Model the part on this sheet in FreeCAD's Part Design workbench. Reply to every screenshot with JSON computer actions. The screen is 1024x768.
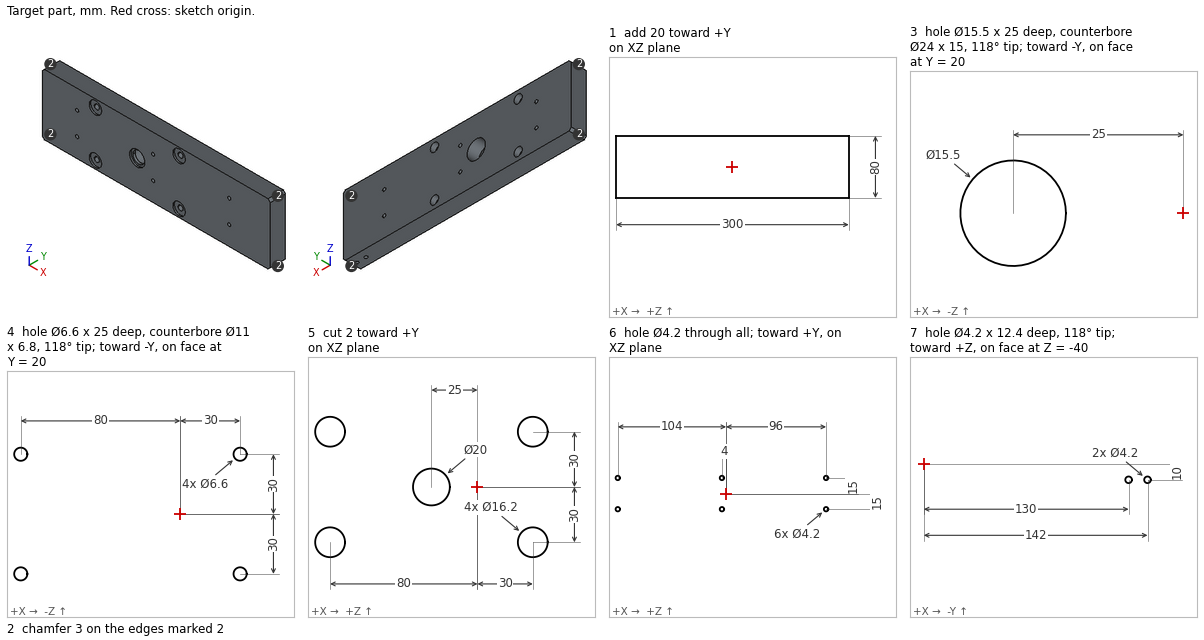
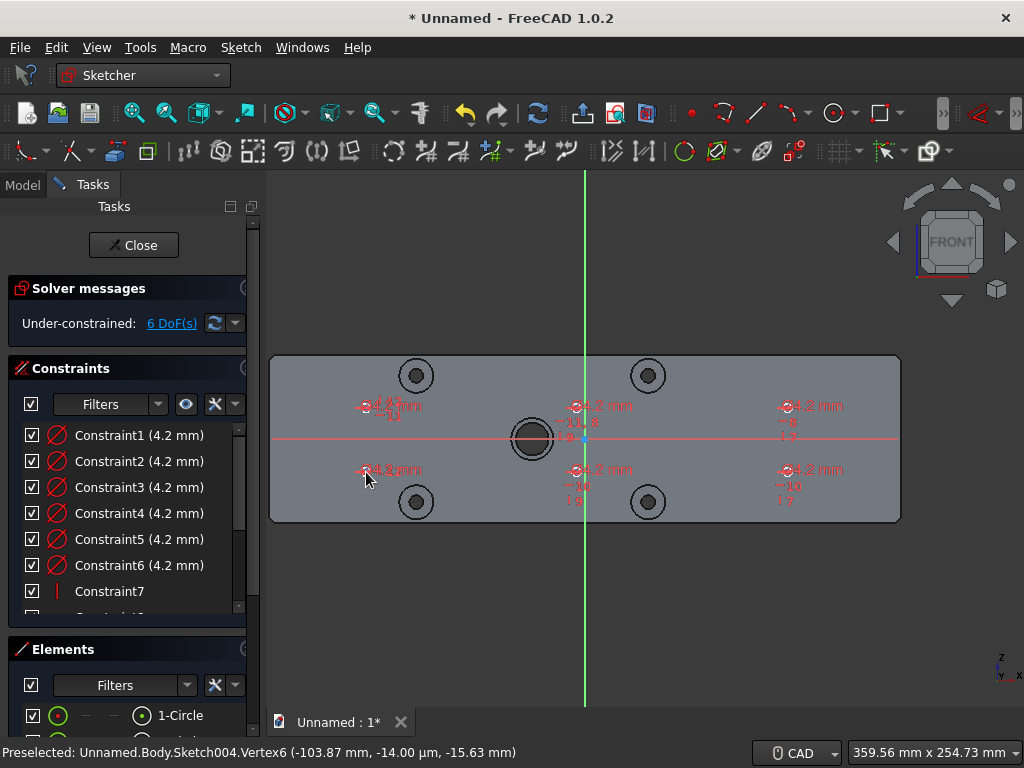
{"action": "left_click", "coordinate": [577, 472]}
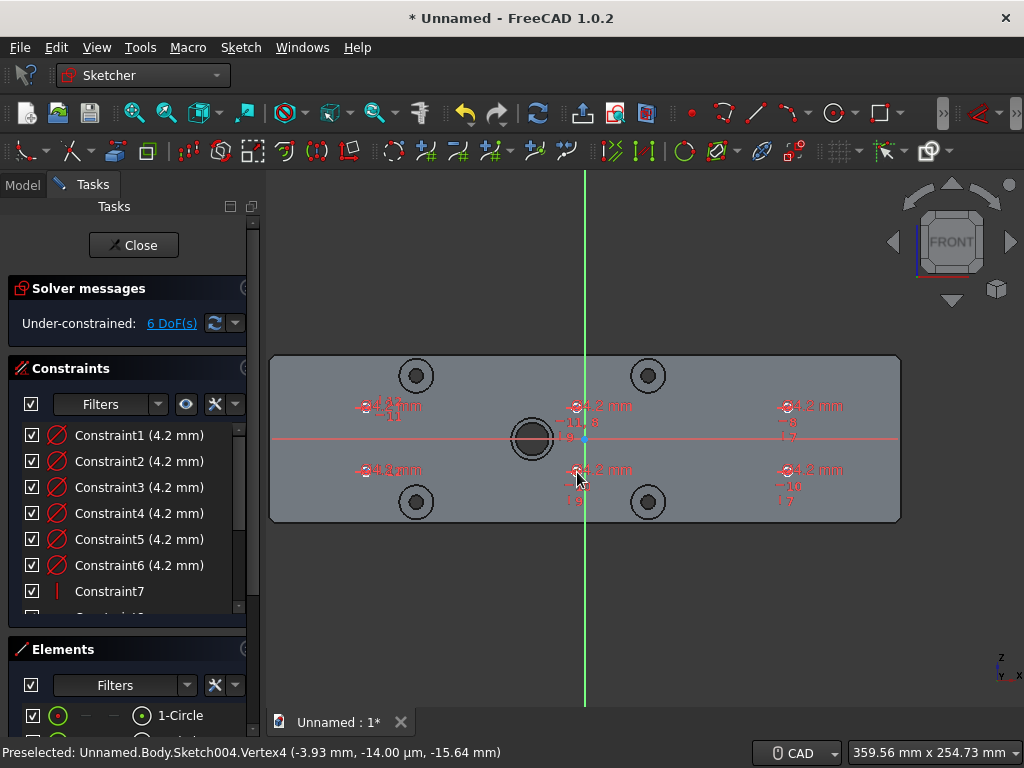
{"action": "left_click", "coordinate": [366, 472]}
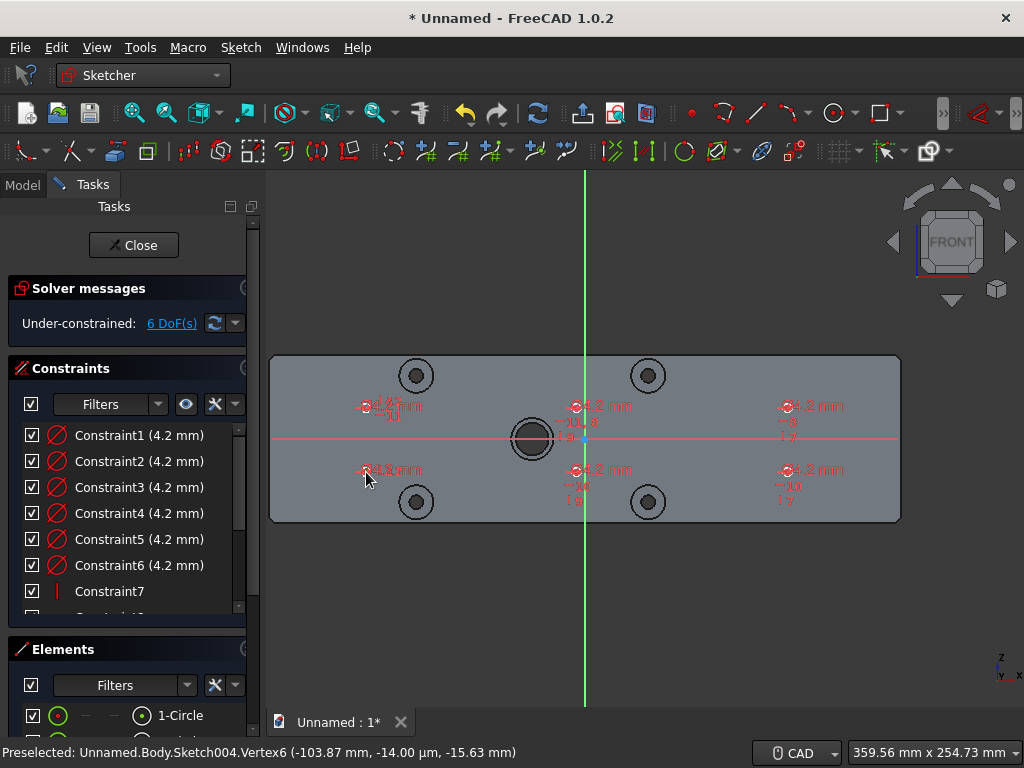
{"action": "key", "text": "h"}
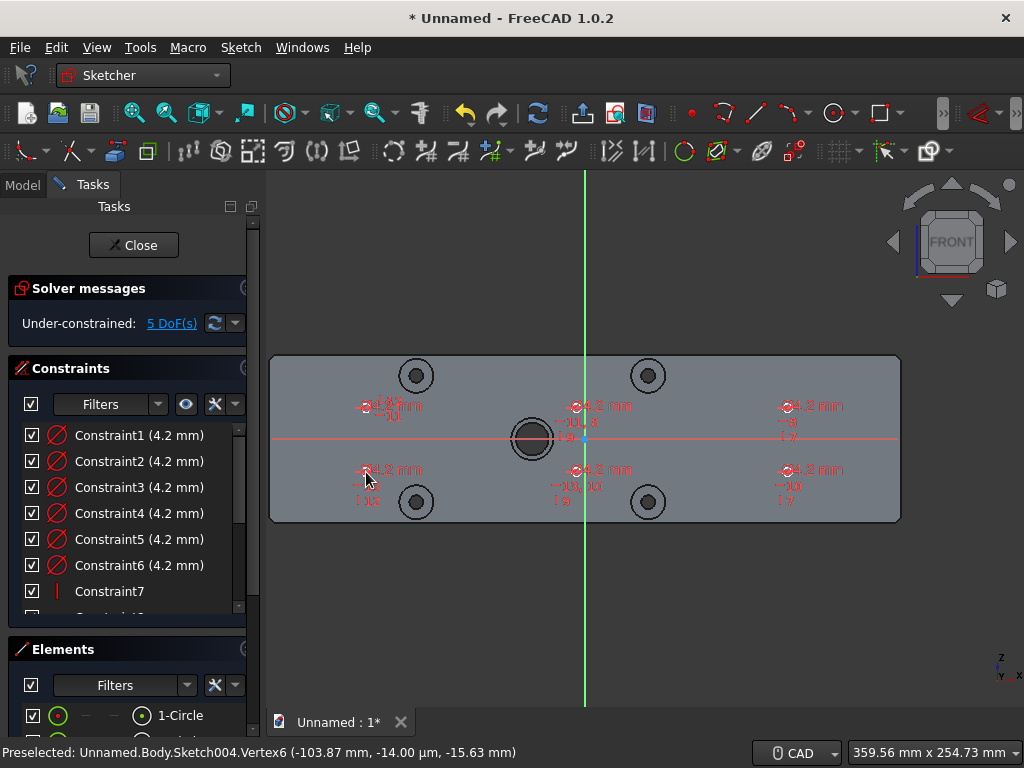
{"action": "left_click", "coordinate": [978, 114]}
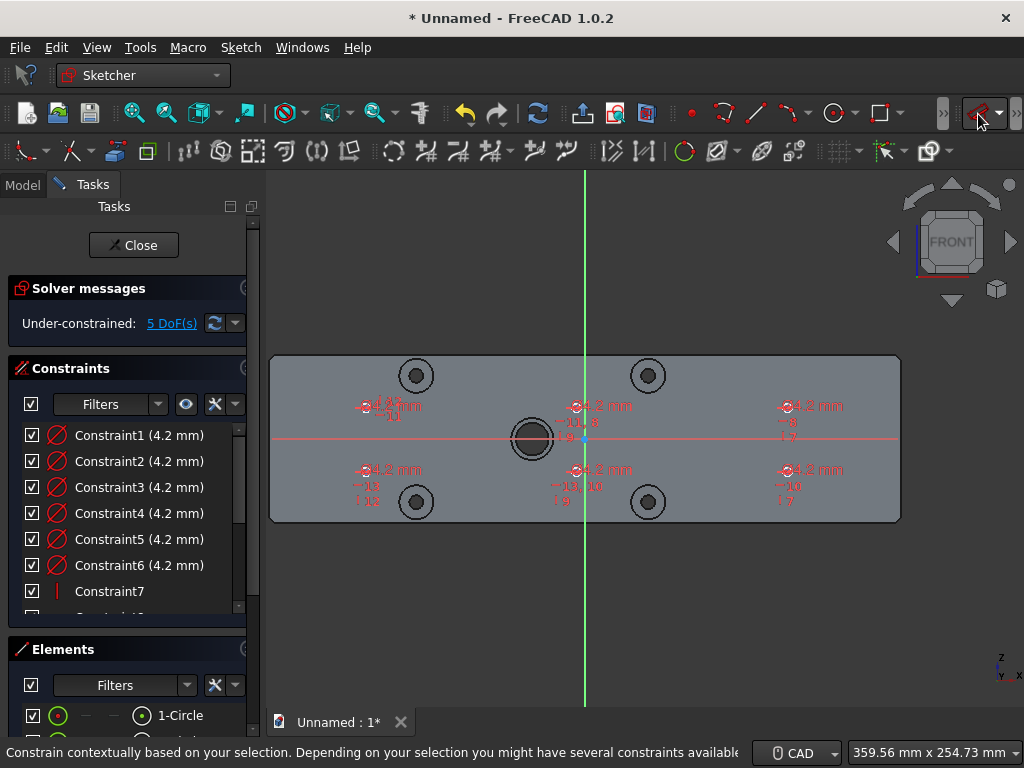
{"action": "scroll", "coordinate": [577, 408], "scroll_direction": "up", "scroll_amount": 8}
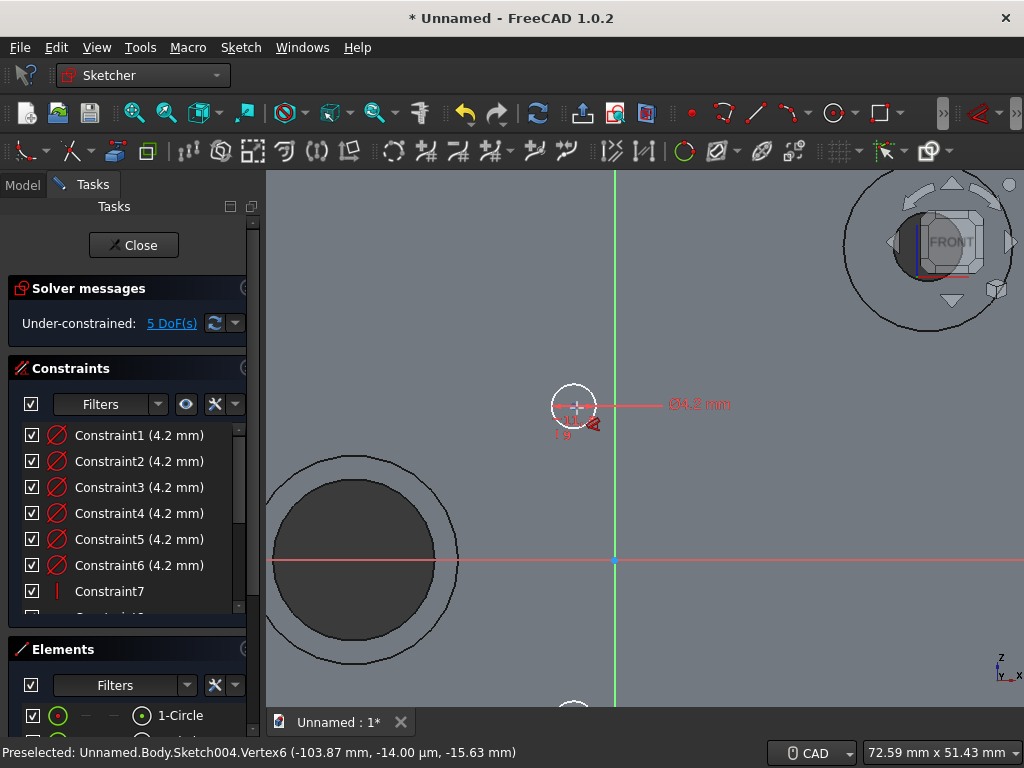
{"action": "left_click", "coordinate": [574, 406]}
{"action": "left_click", "coordinate": [594, 372]}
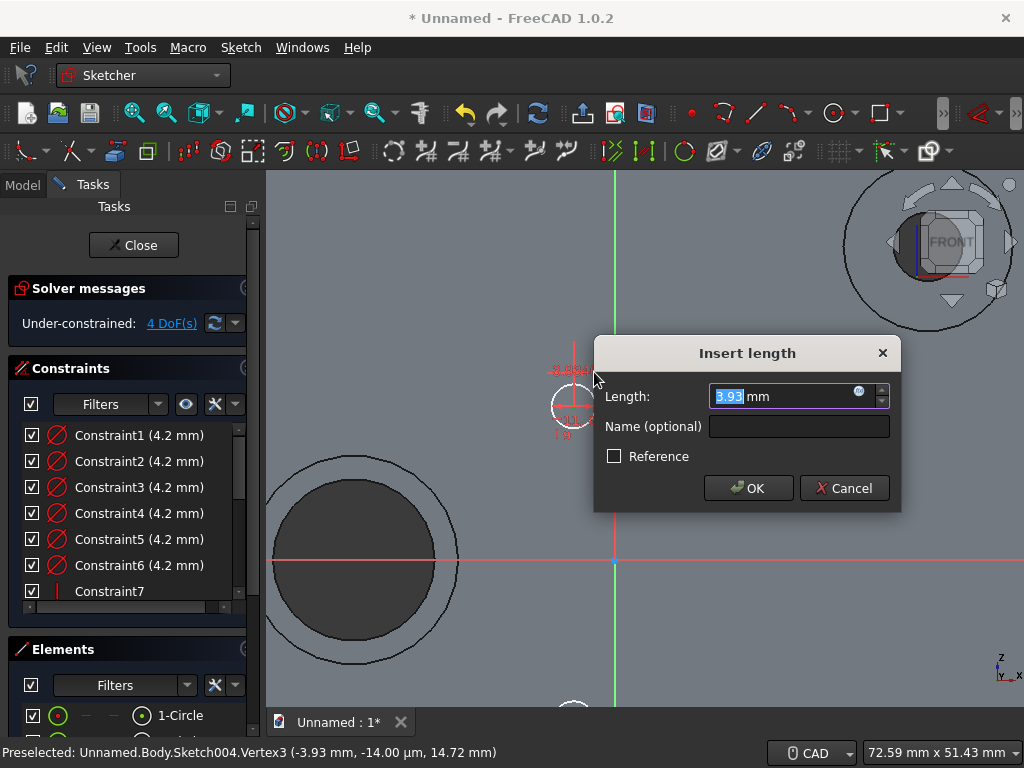
{"action": "type", "text": "4"}
{"action": "key", "text": "Return"}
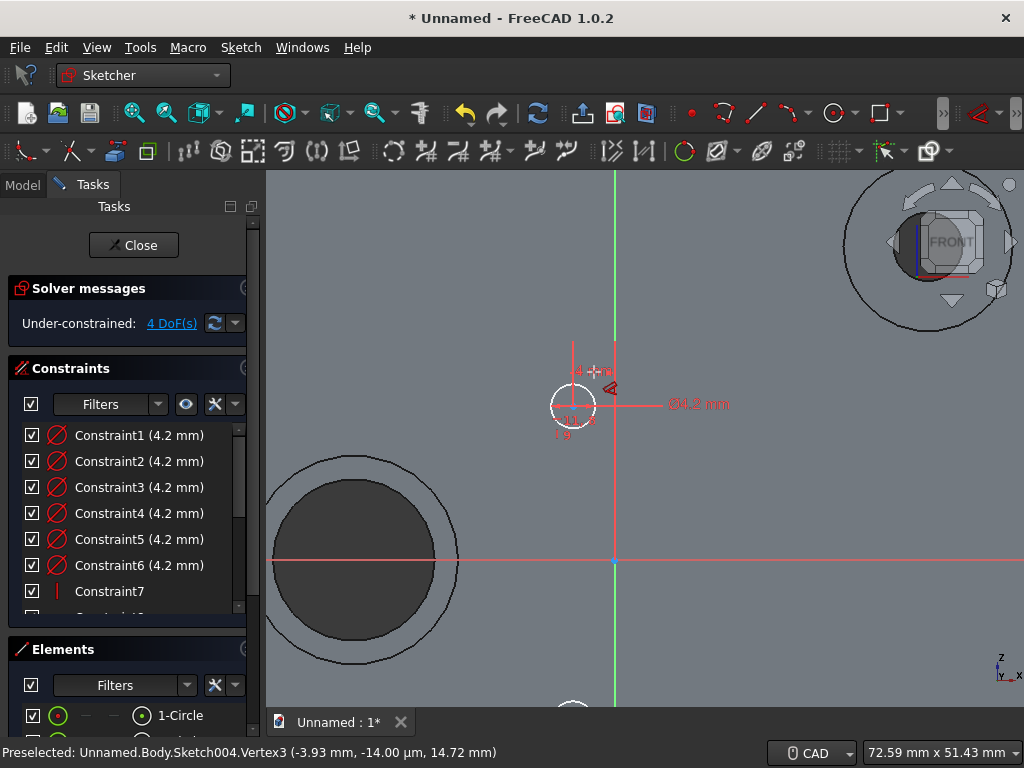
{"action": "scroll", "coordinate": [577, 408], "scroll_direction": "down", "scroll_amount": 8}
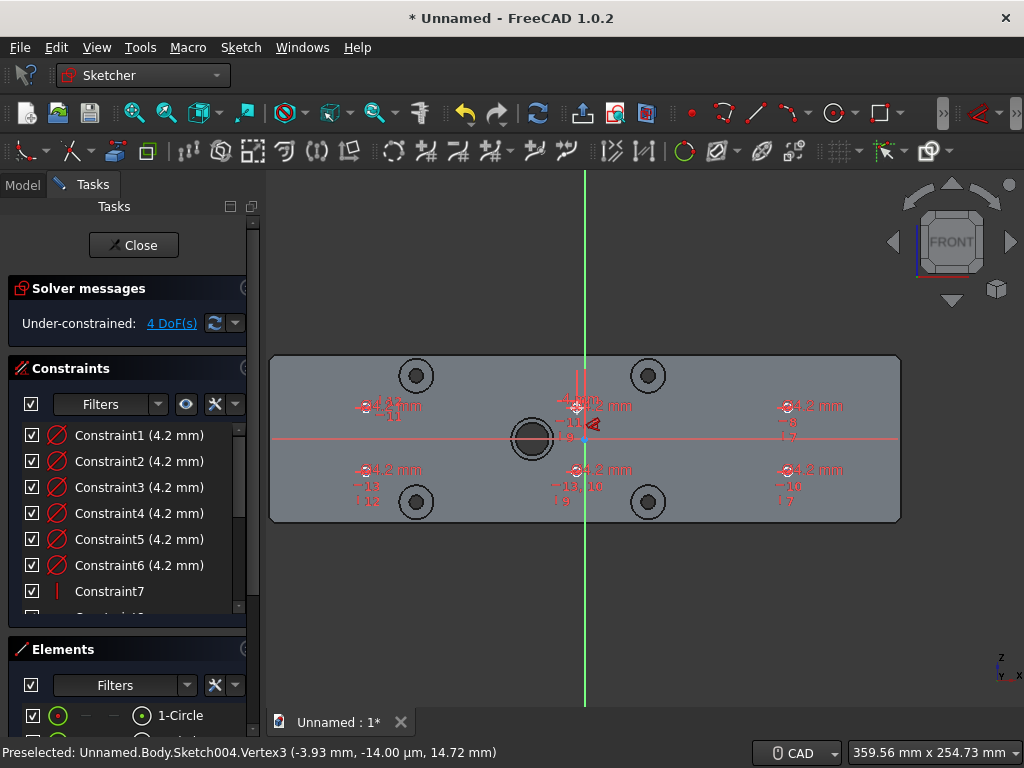
{"action": "left_click", "coordinate": [787, 408]}
{"action": "left_click", "coordinate": [686, 374]}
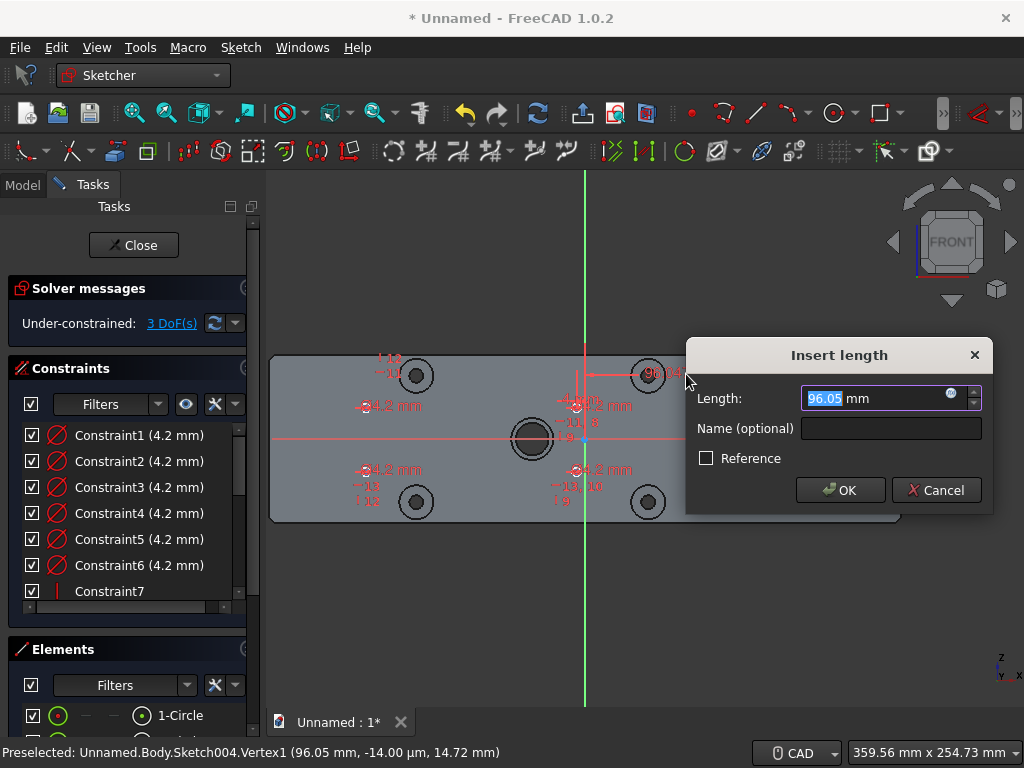
{"action": "type", "text": "96"}
{"action": "key", "text": "Return"}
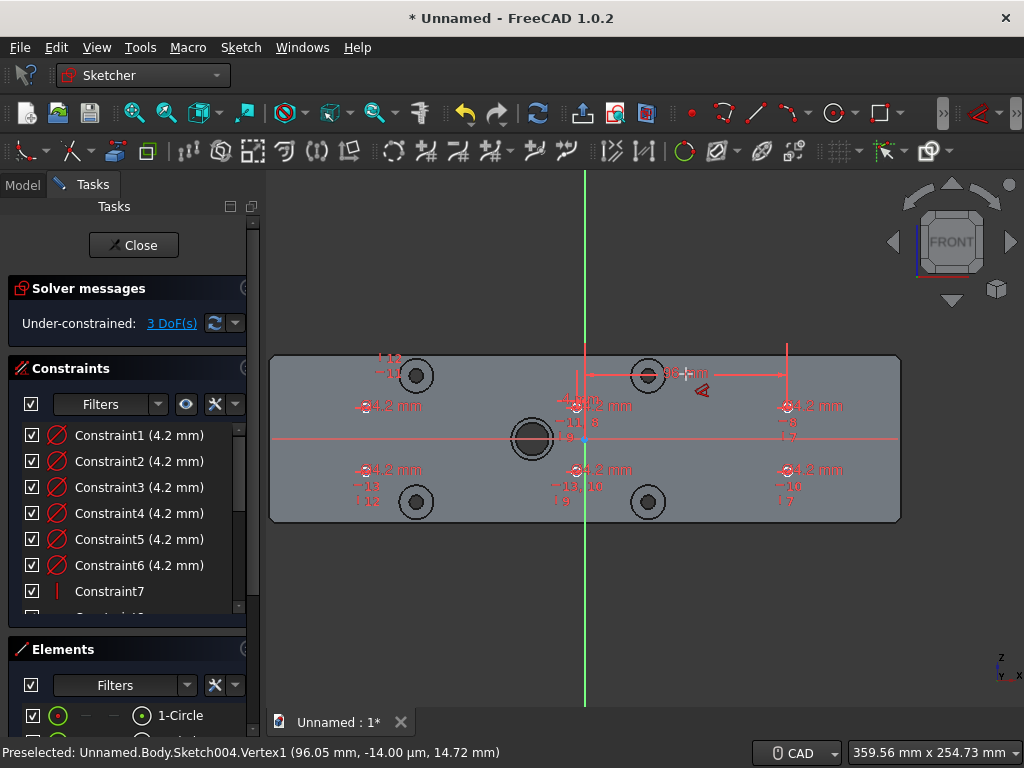
{"action": "scroll", "coordinate": [787, 408], "scroll_direction": "up", "scroll_amount": 2}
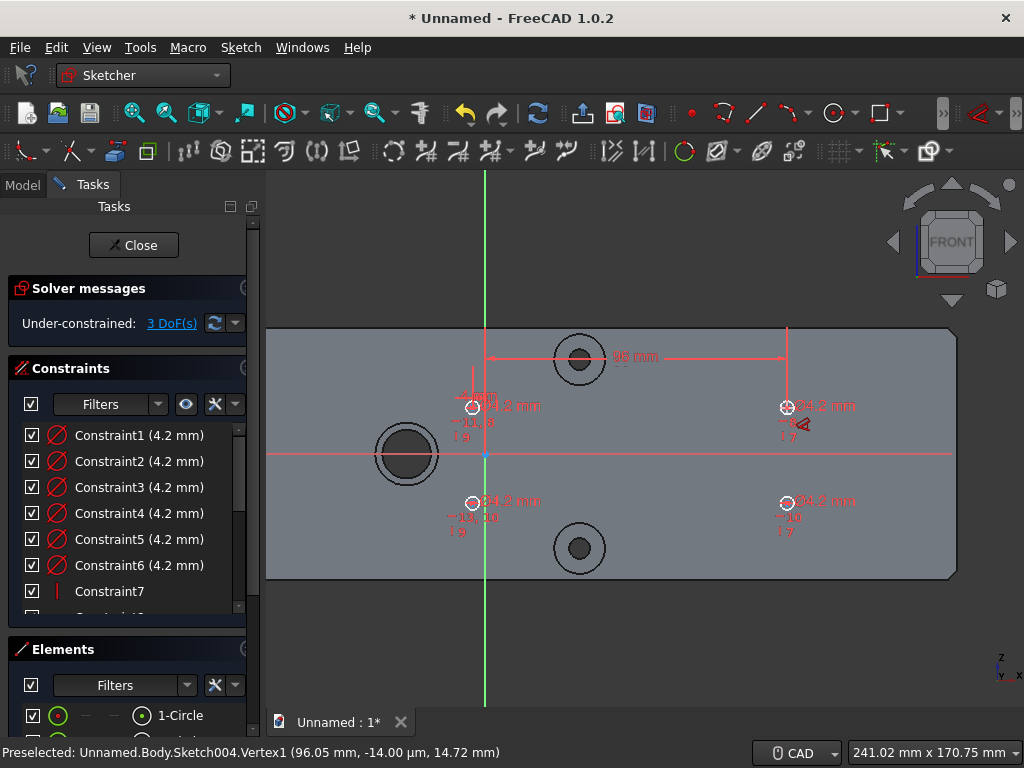
{"action": "left_click", "coordinate": [787, 408]}
{"action": "left_click", "coordinate": [821, 431]}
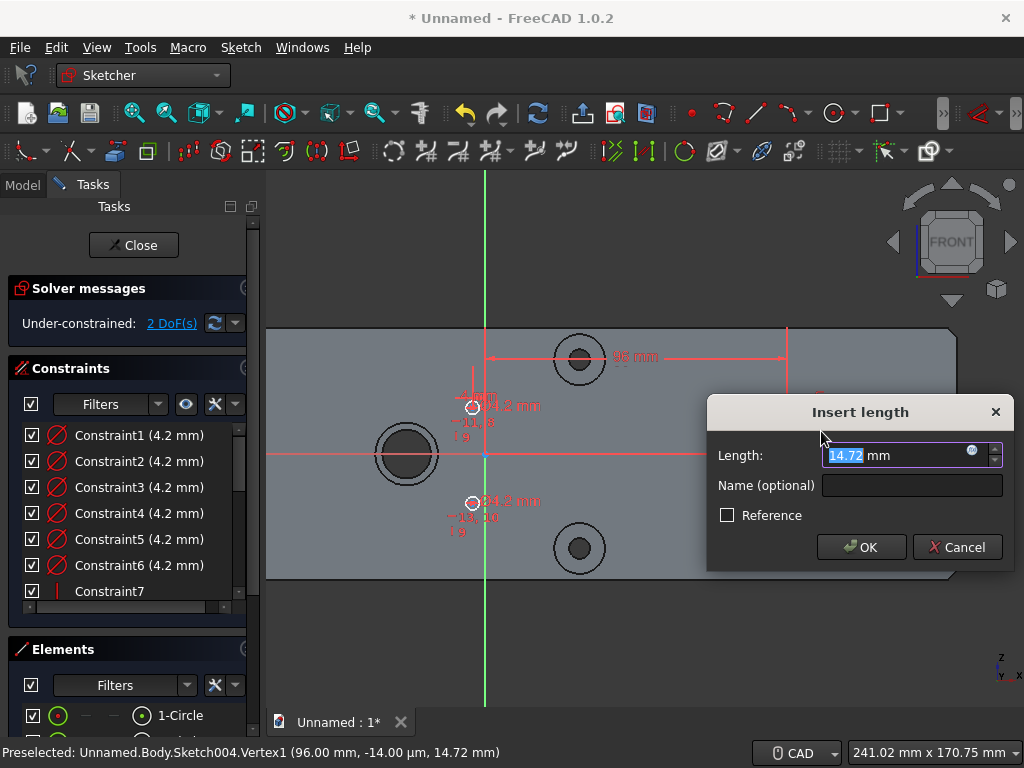
{"action": "type", "text": "15"}
{"action": "key", "text": "Return"}